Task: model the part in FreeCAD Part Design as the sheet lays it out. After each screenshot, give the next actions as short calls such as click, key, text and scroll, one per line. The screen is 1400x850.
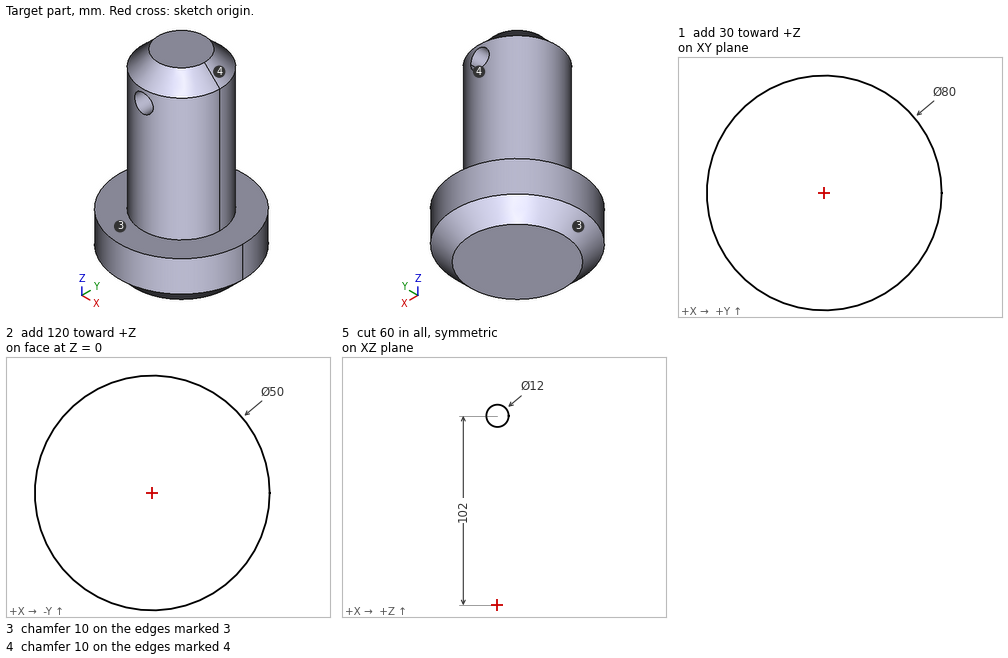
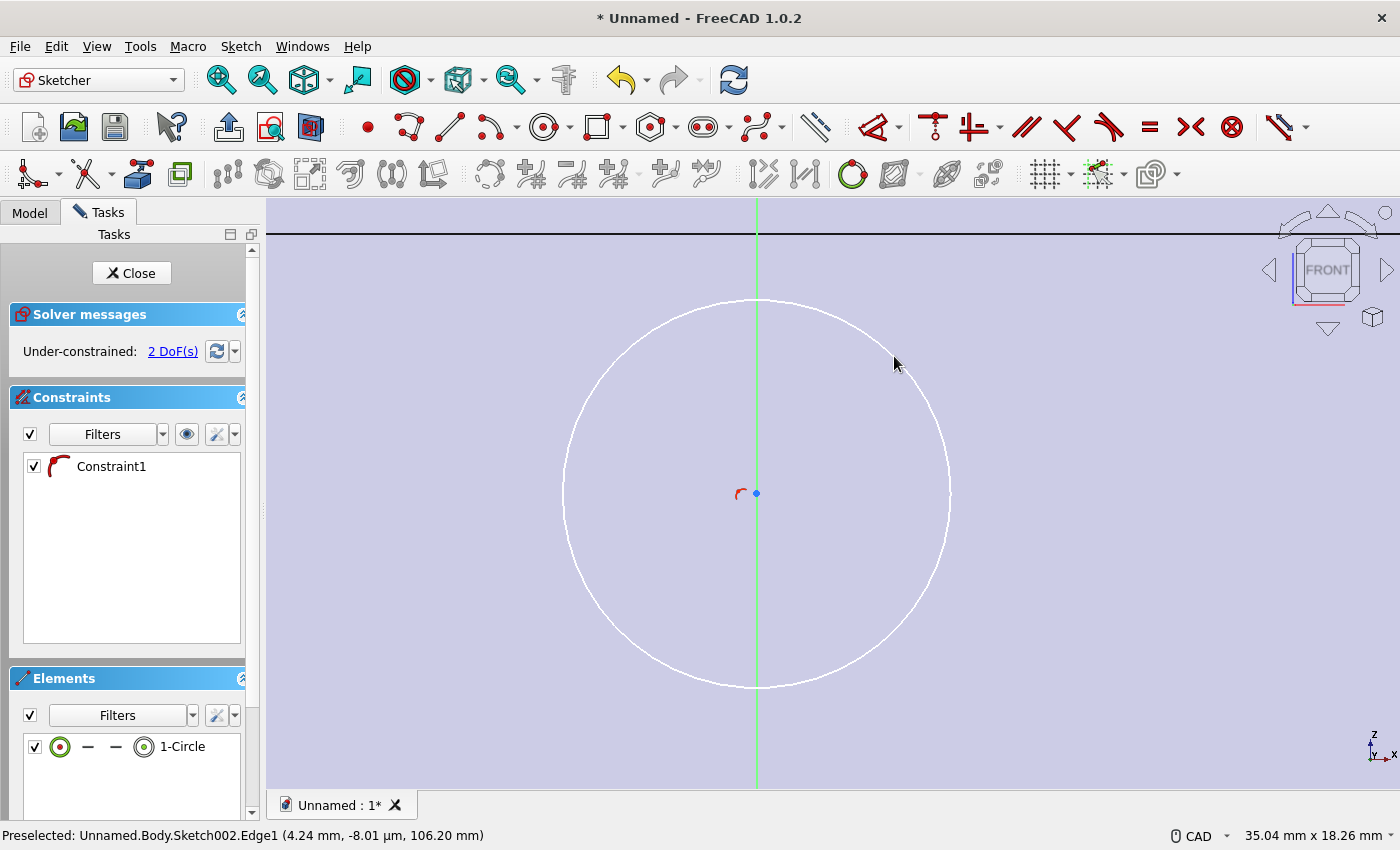
click(872, 128)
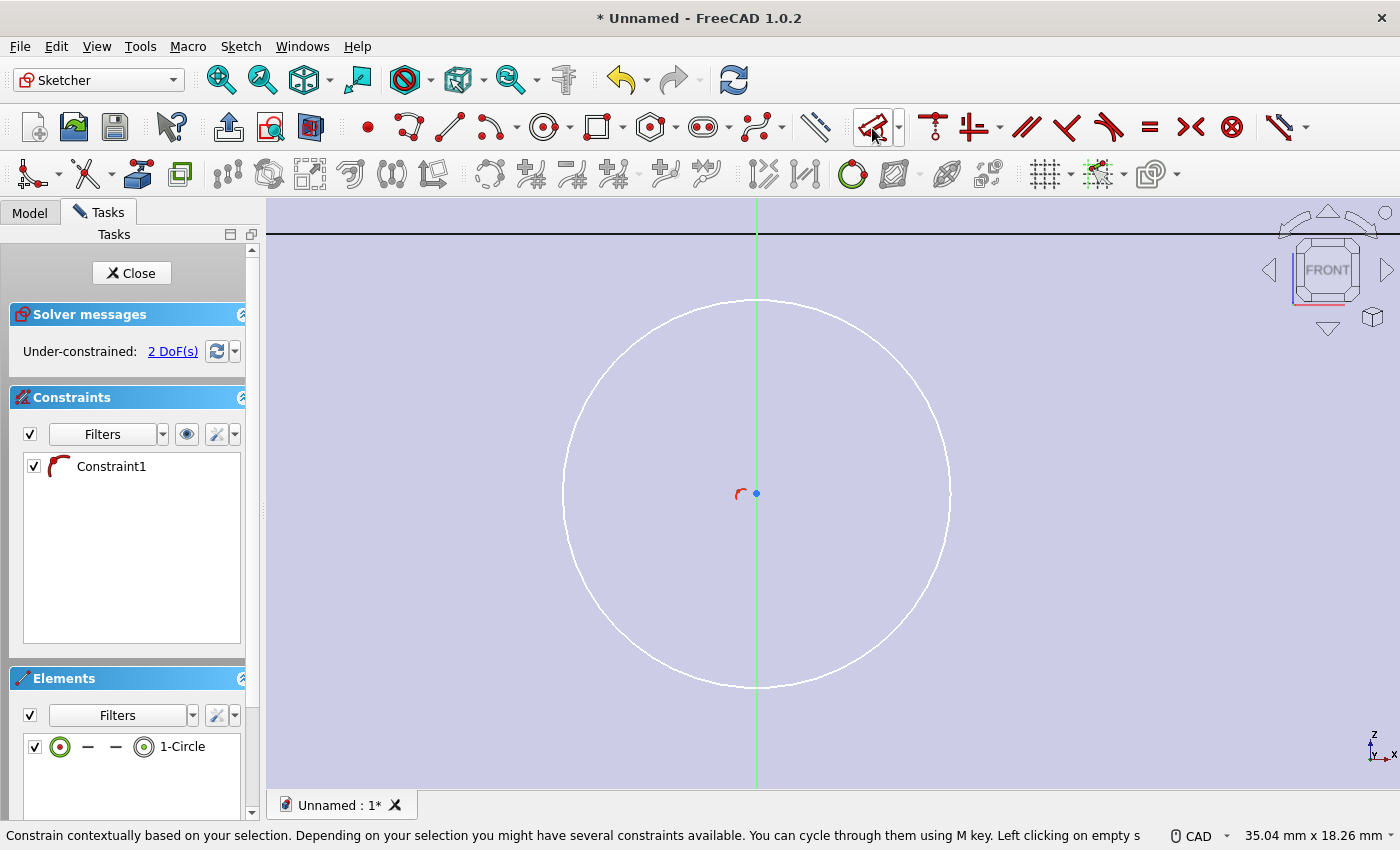
click(893, 356)
click(915, 333)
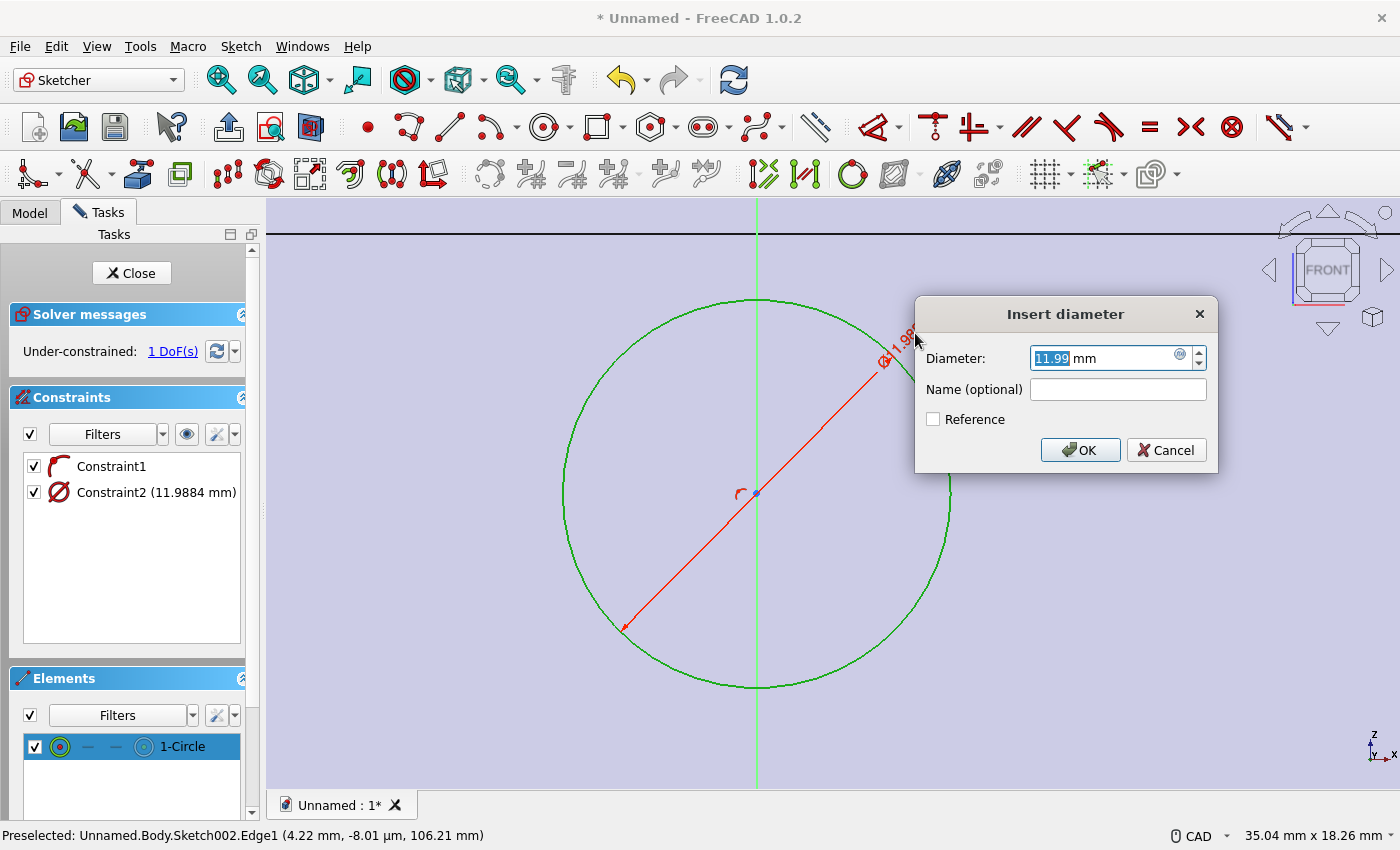
text(12)
key(Return)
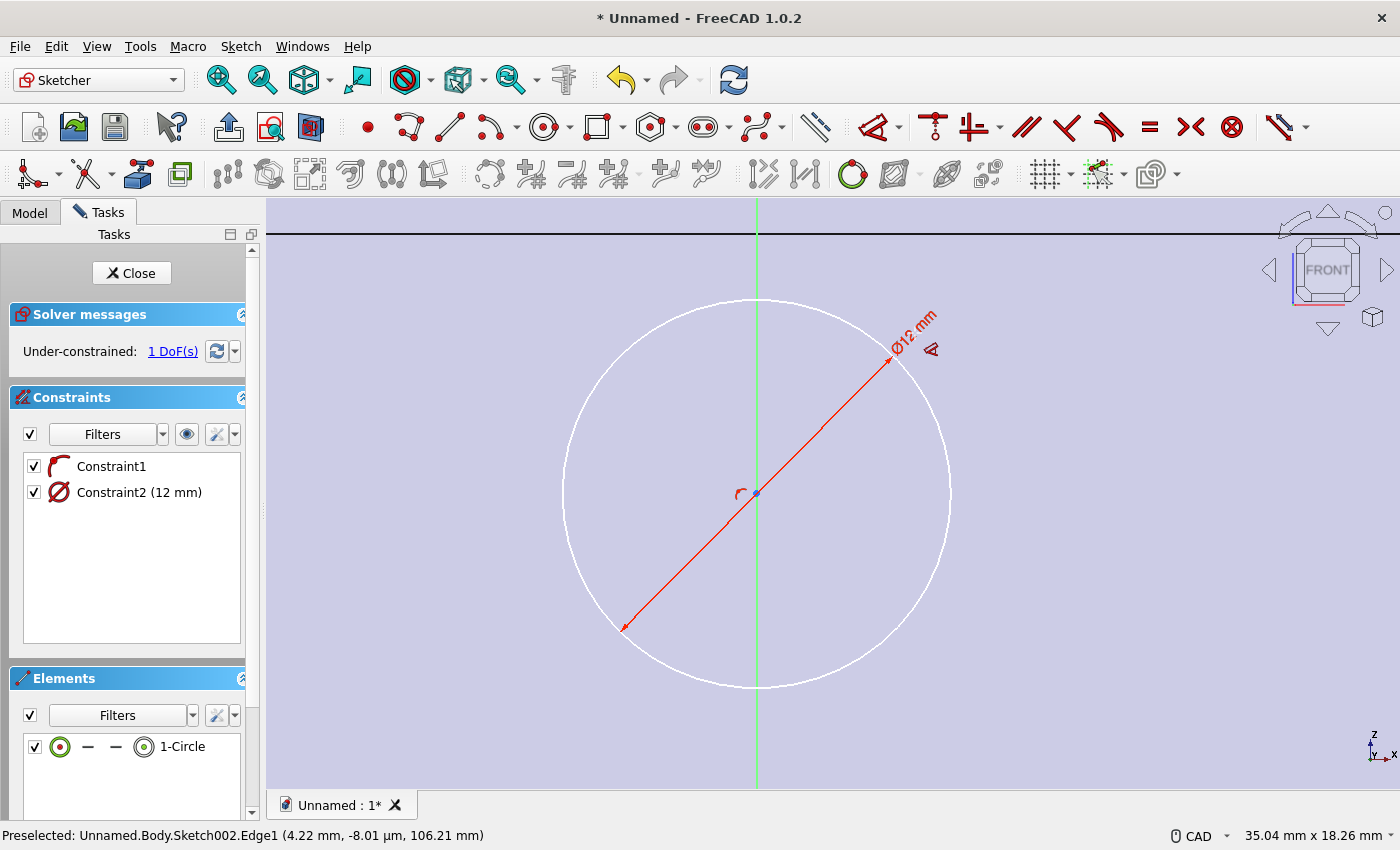
click(757, 494)
click(791, 627)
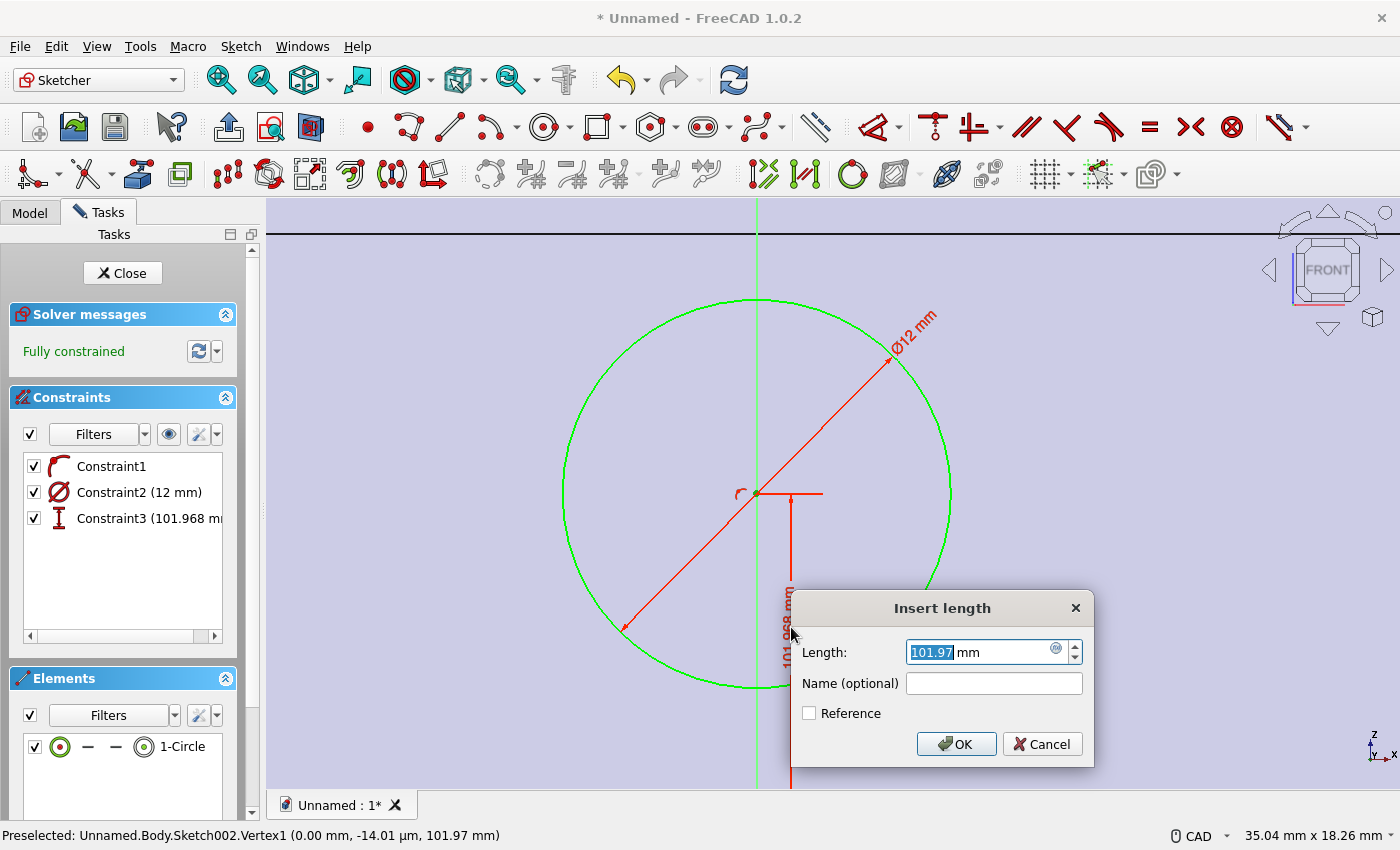
text(102)
key(Return)
key(Escape)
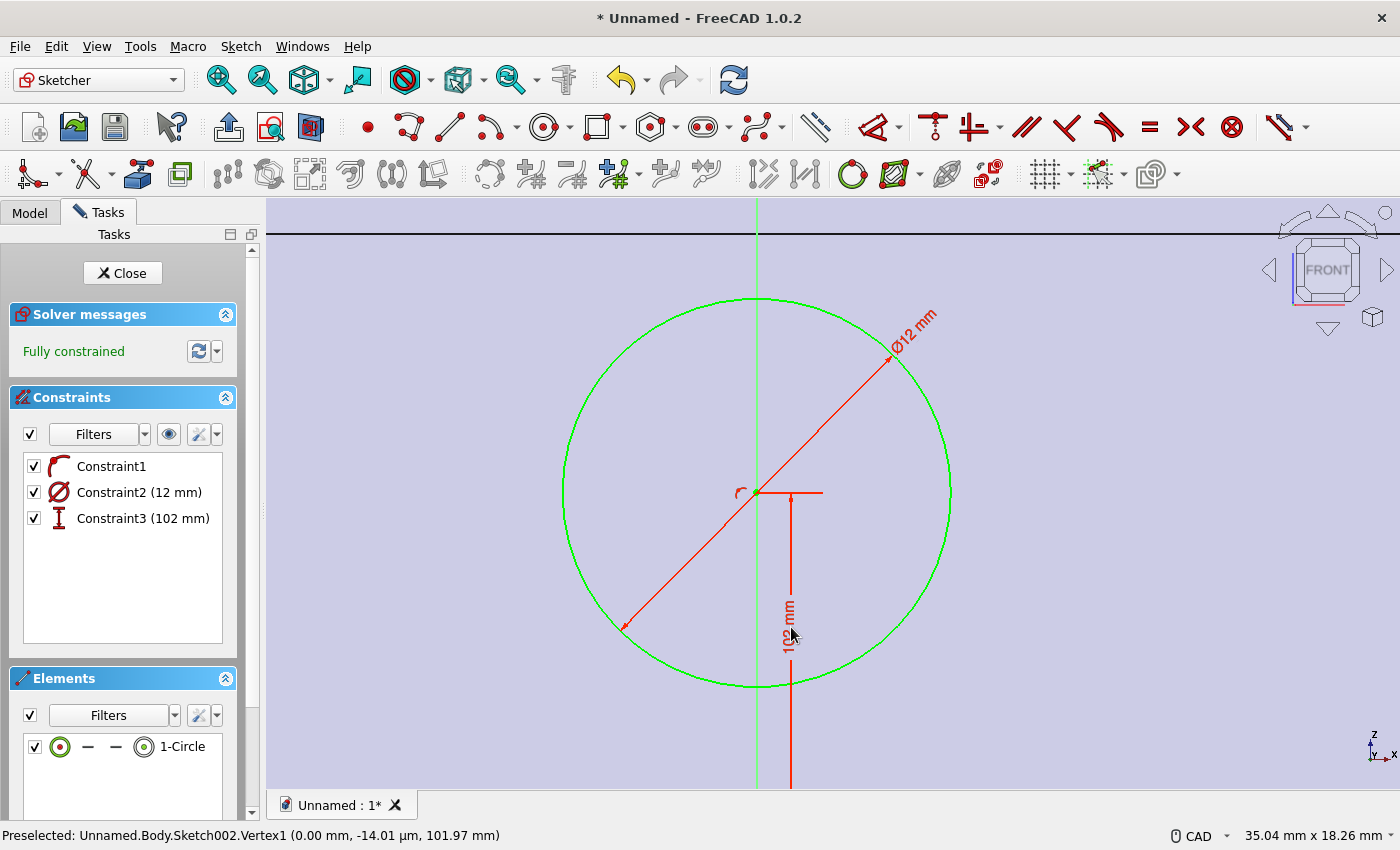
click(123, 273)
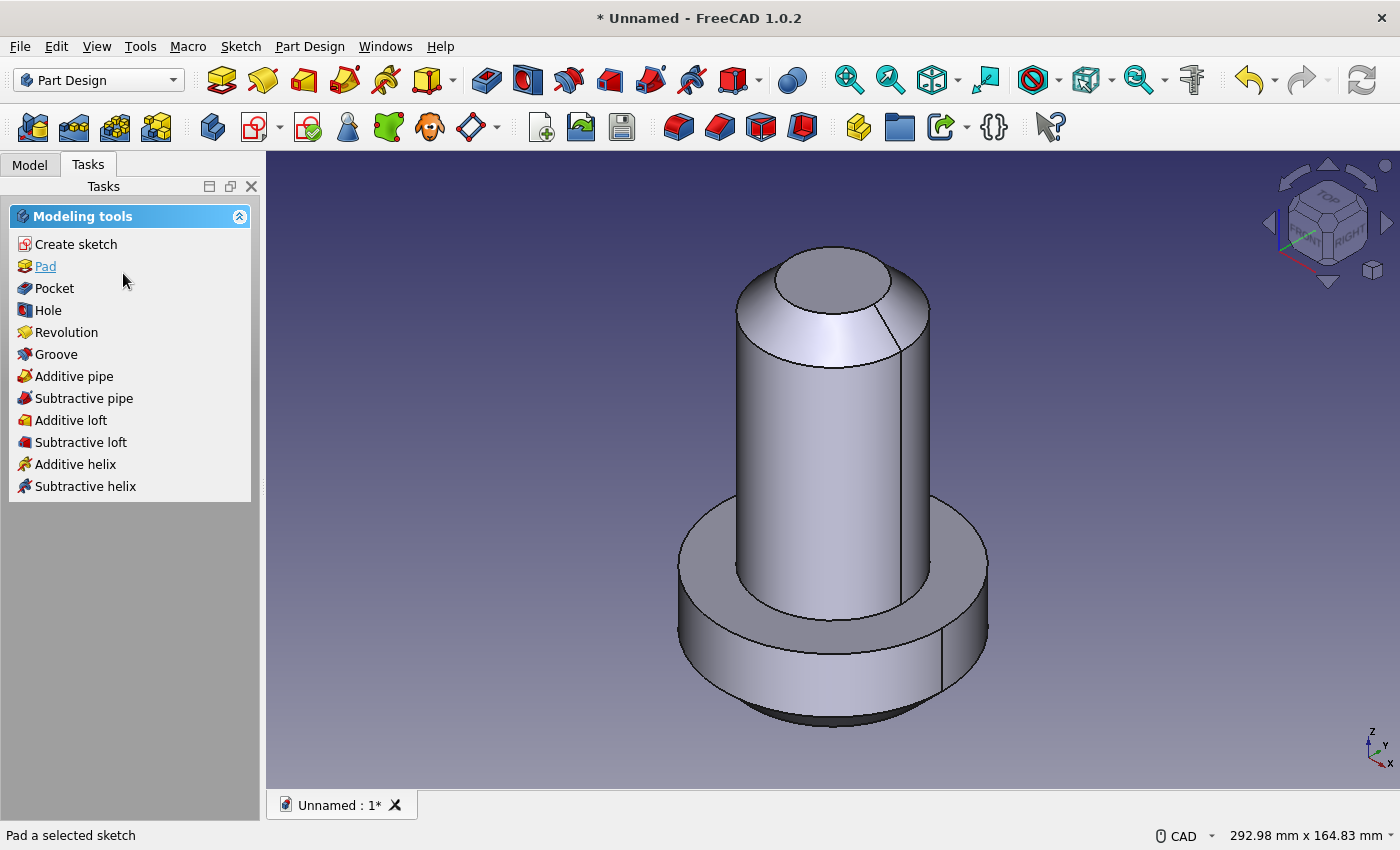
click(487, 80)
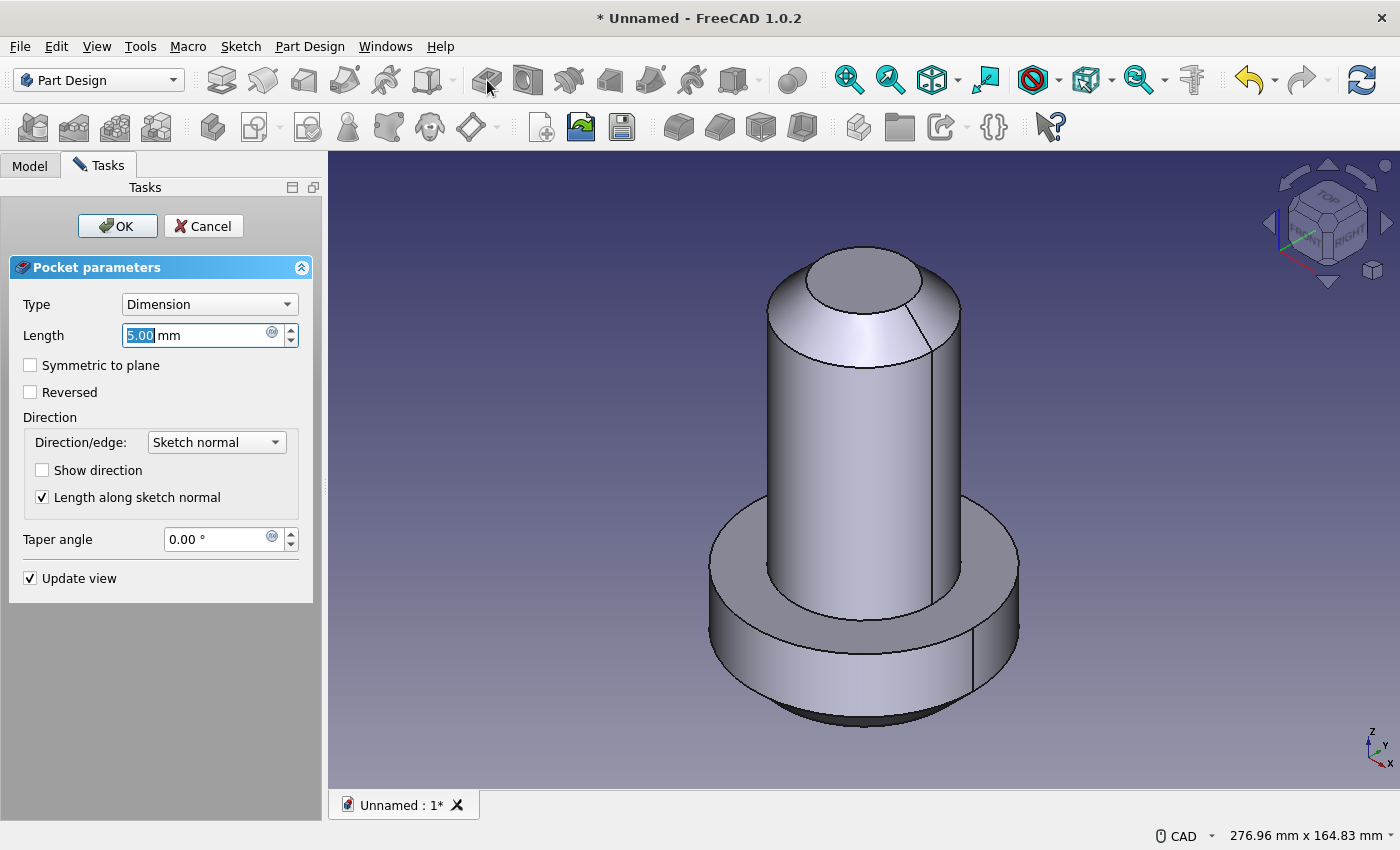
text(60)
key(Tab)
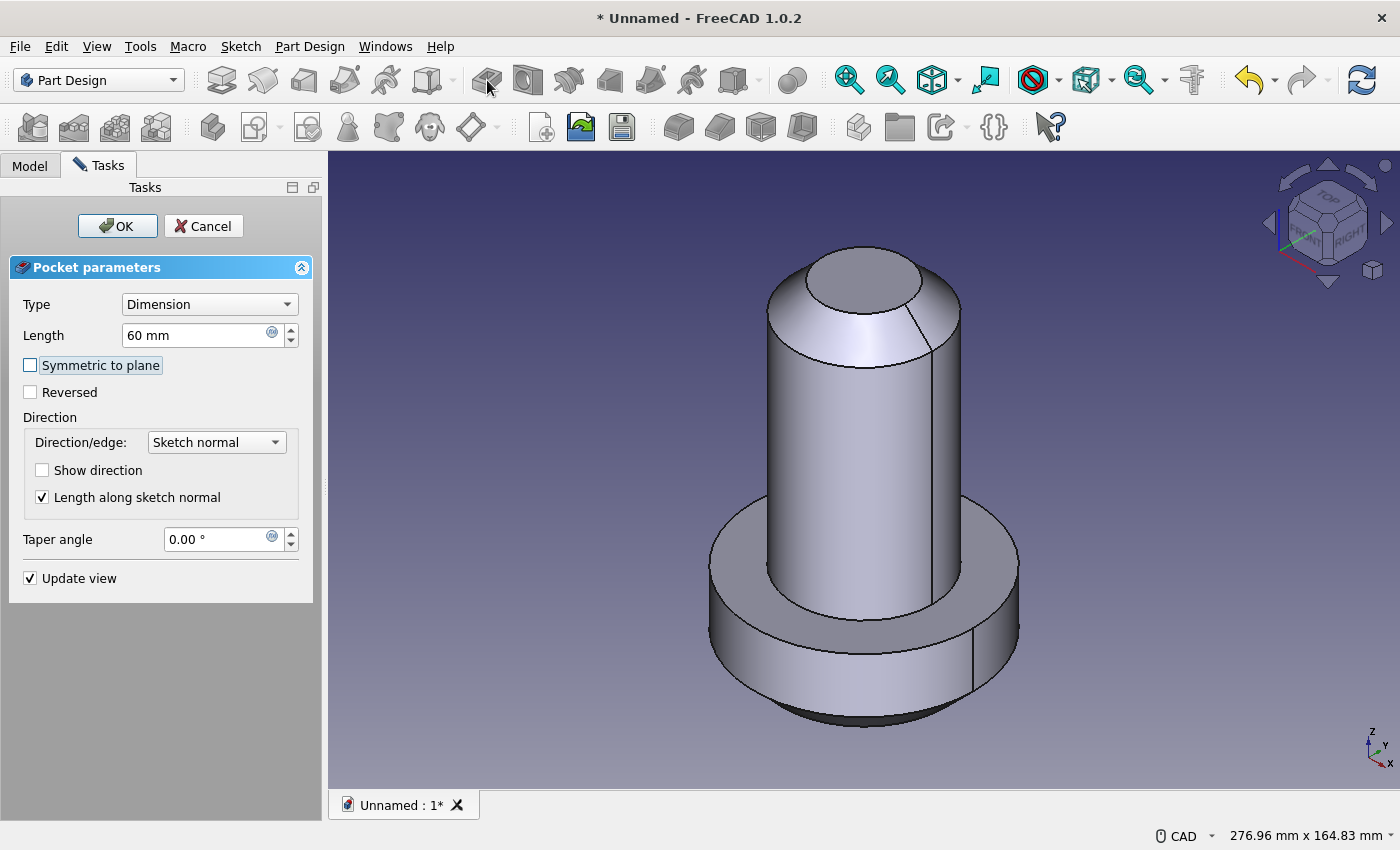
click(31, 365)